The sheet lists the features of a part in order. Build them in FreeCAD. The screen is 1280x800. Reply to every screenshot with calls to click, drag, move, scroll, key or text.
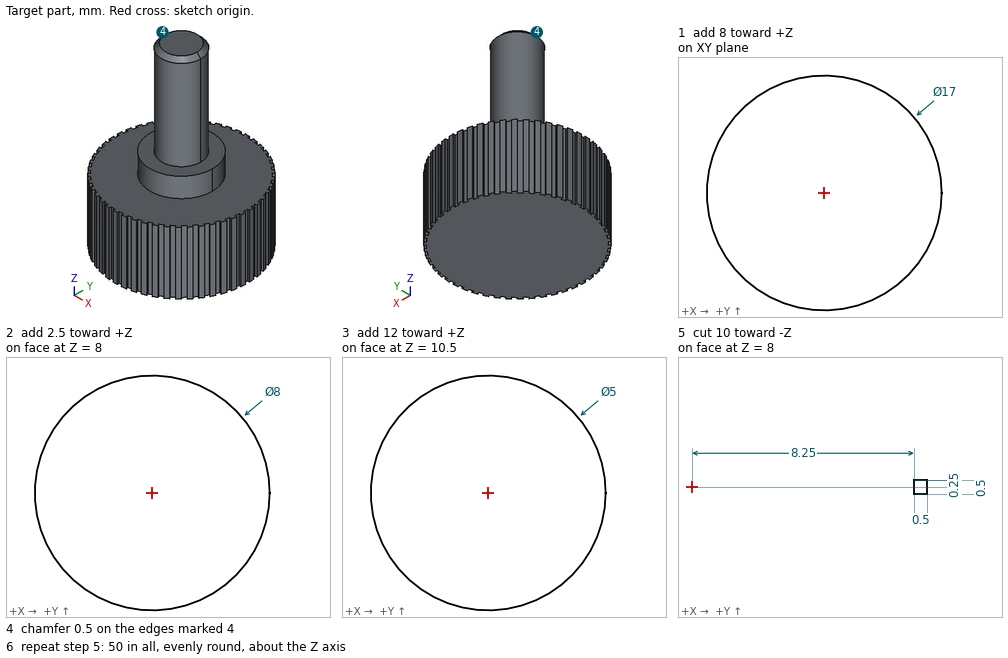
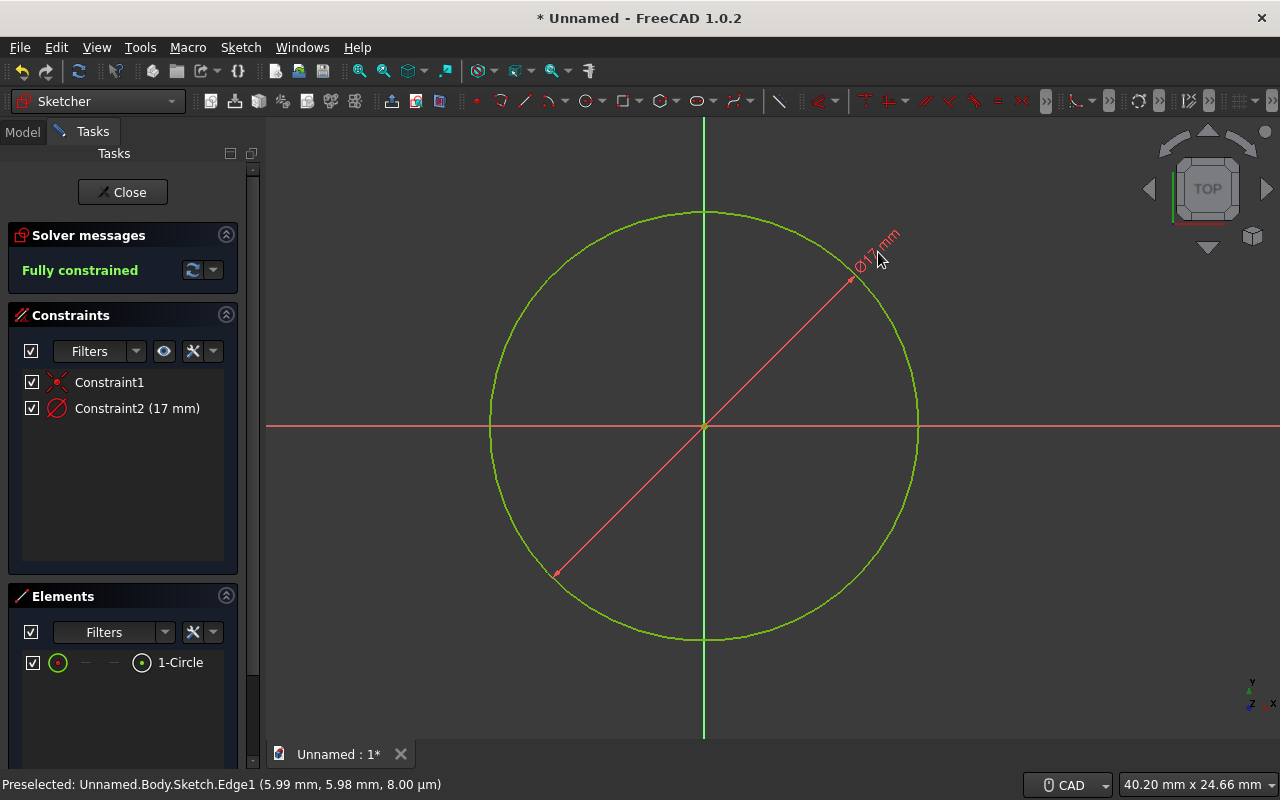
click(123, 192)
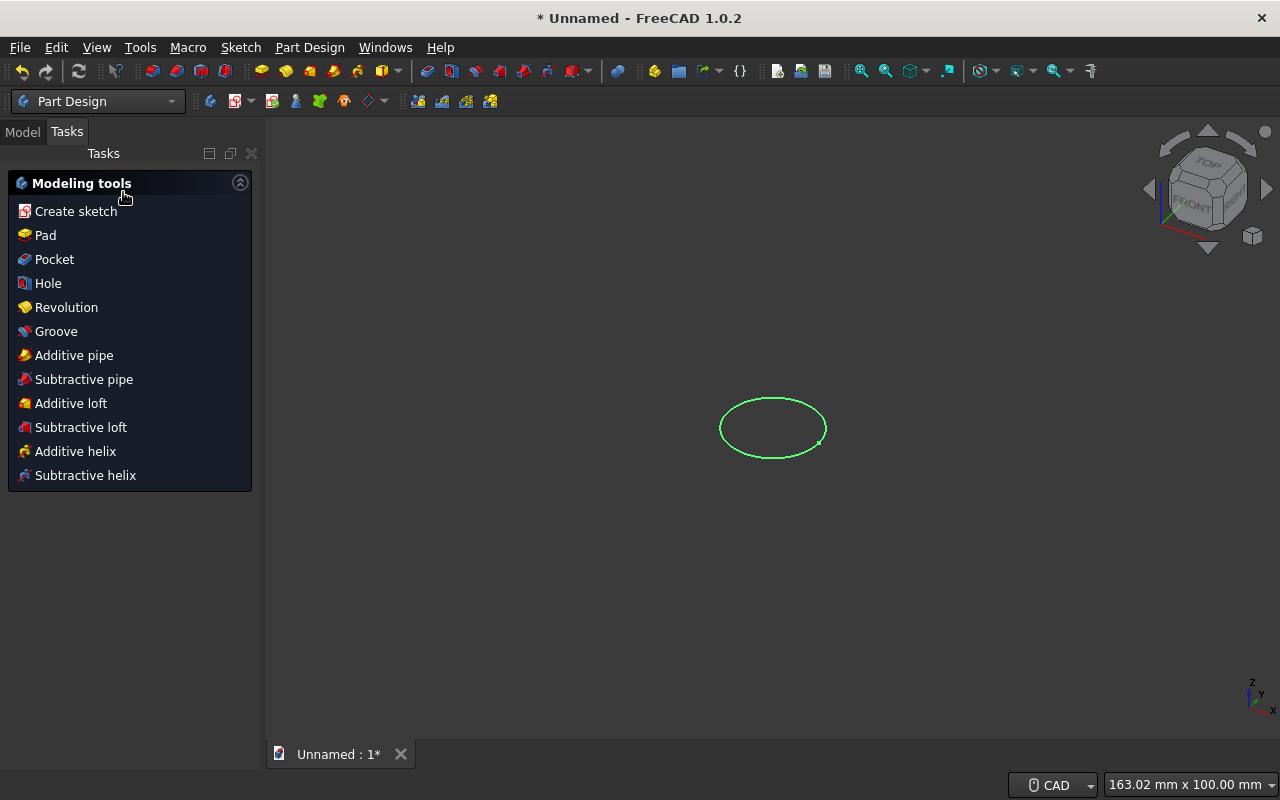
click(262, 72)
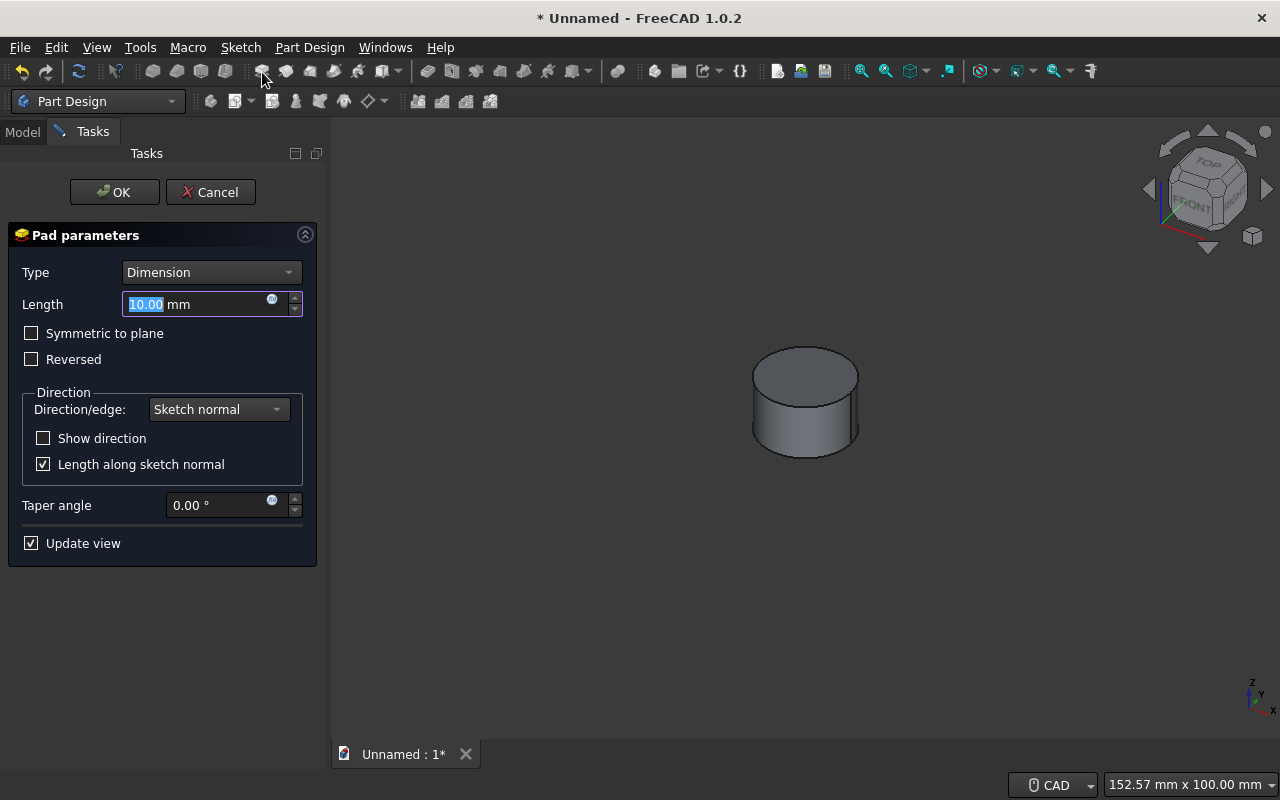
text(8)
key(Tab)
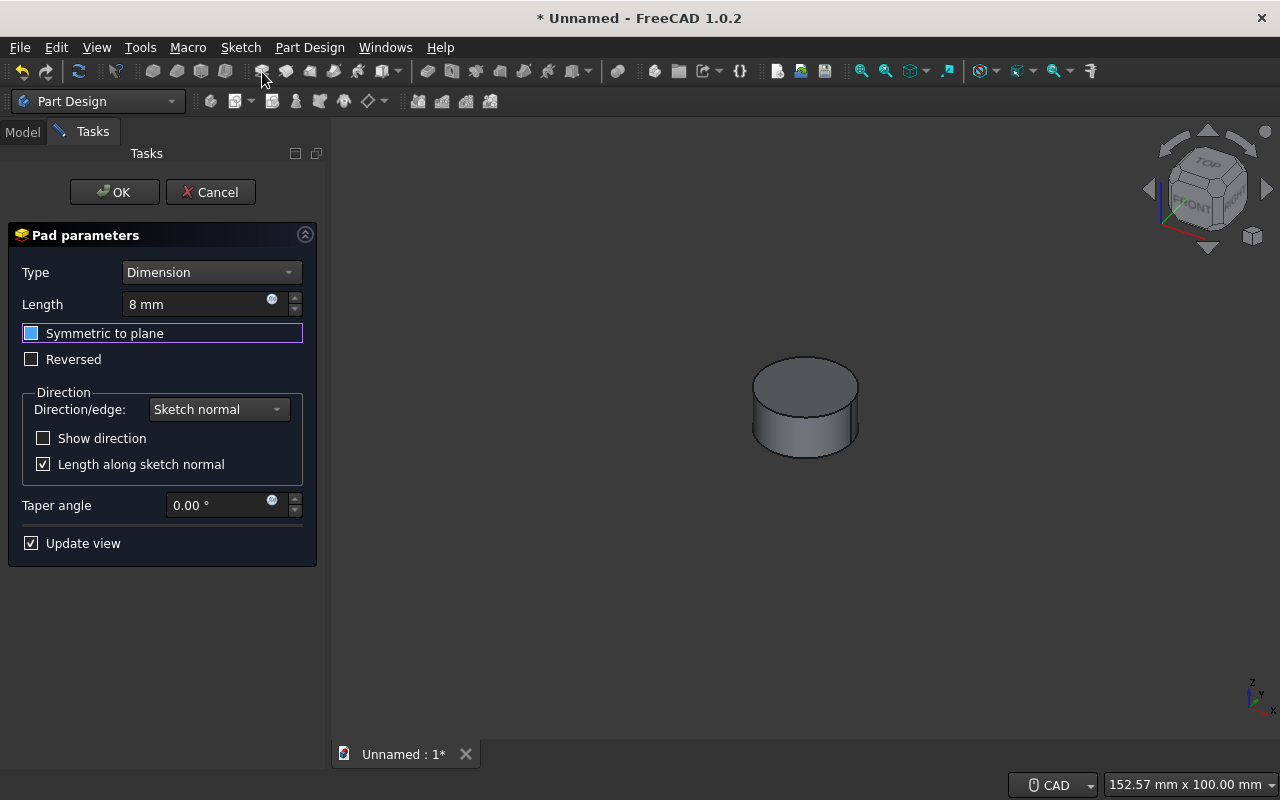
click(115, 192)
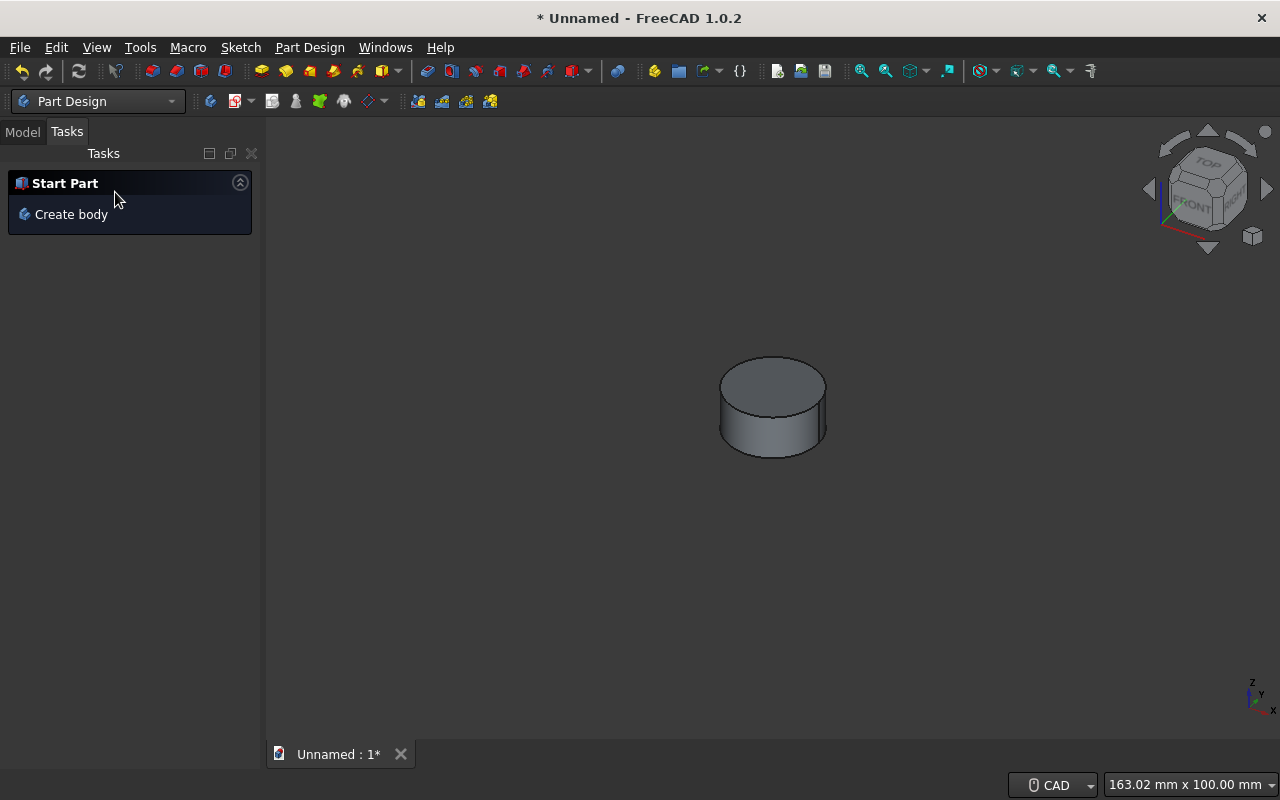
key(v)
key(f)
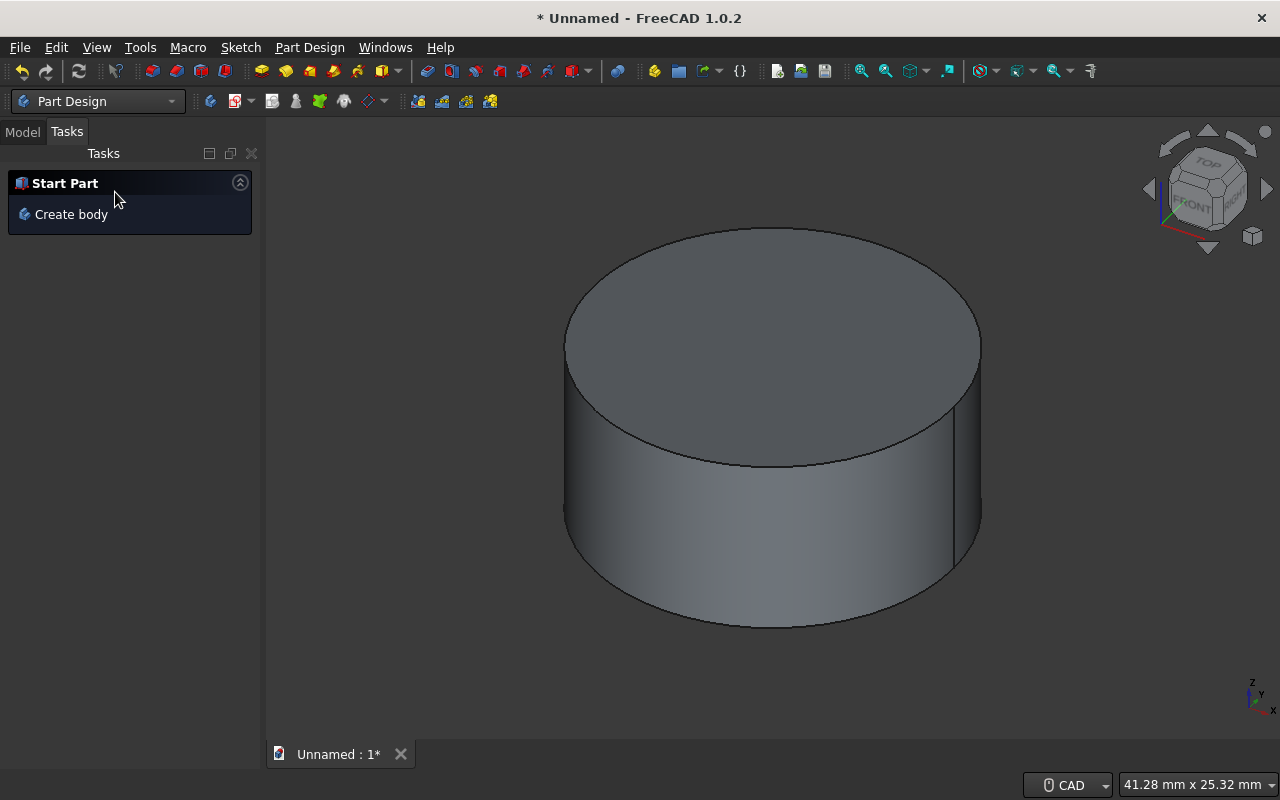
click(773, 346)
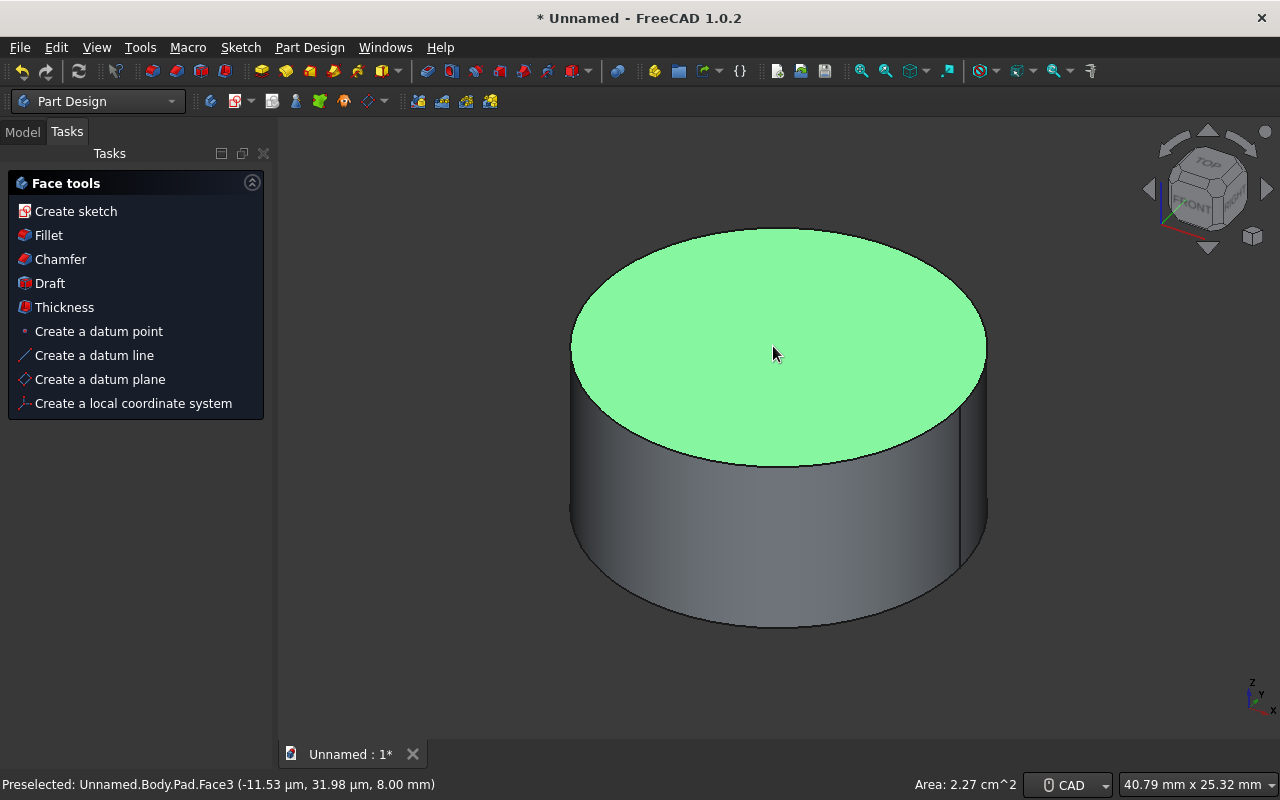
click(236, 102)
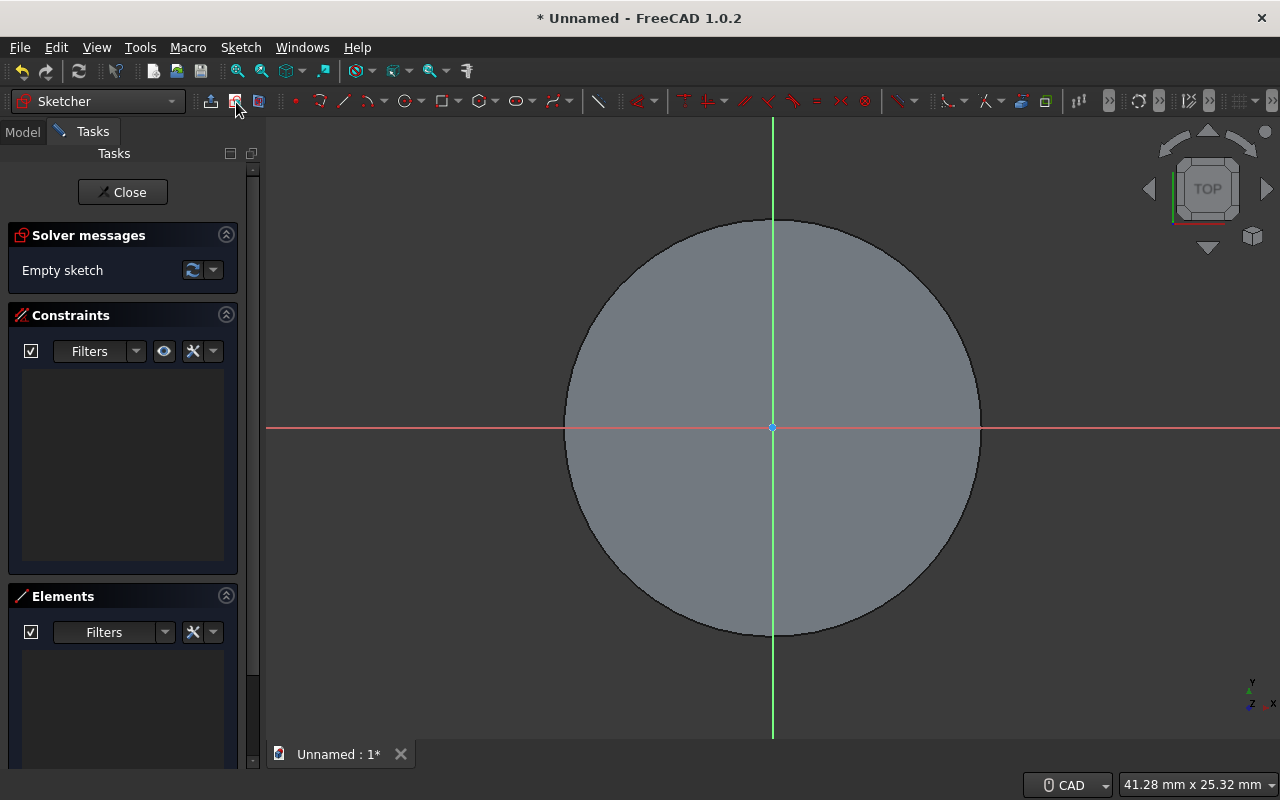
scroll(829, 428, up, 4)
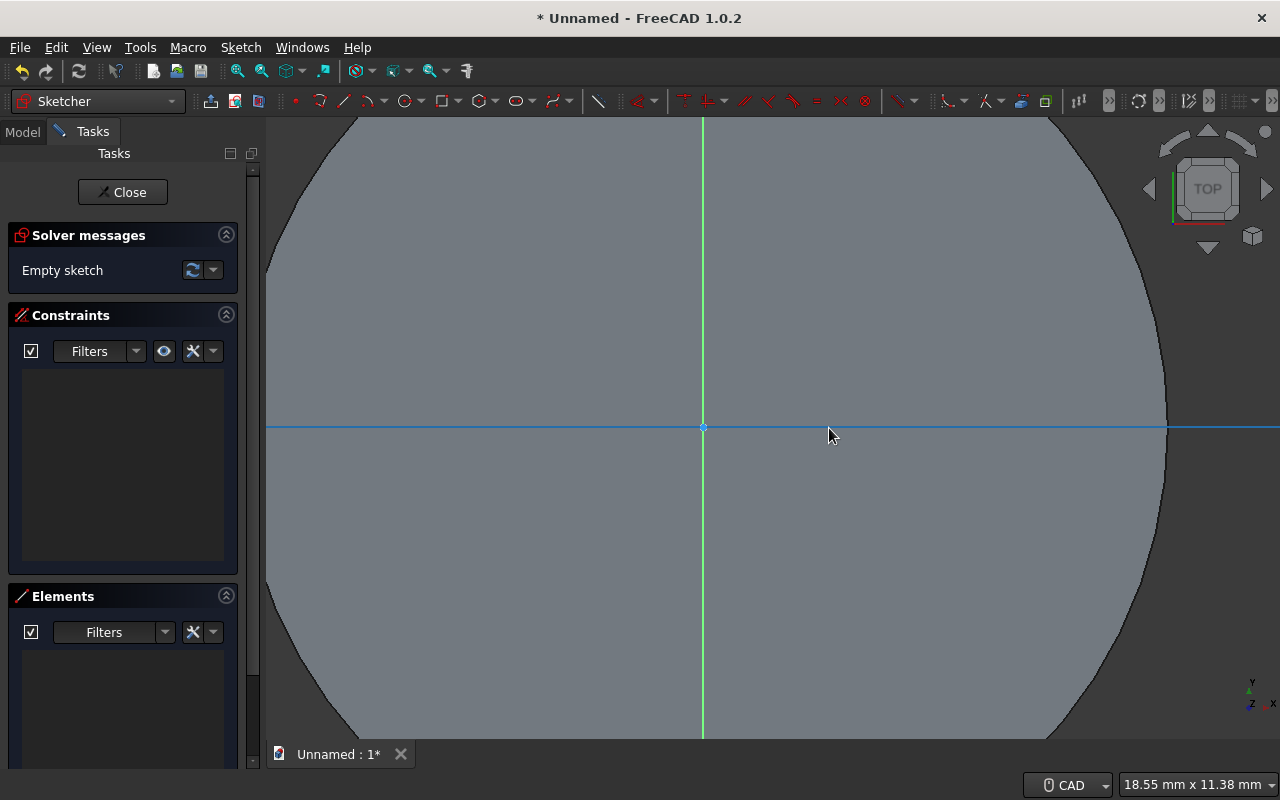
click(406, 102)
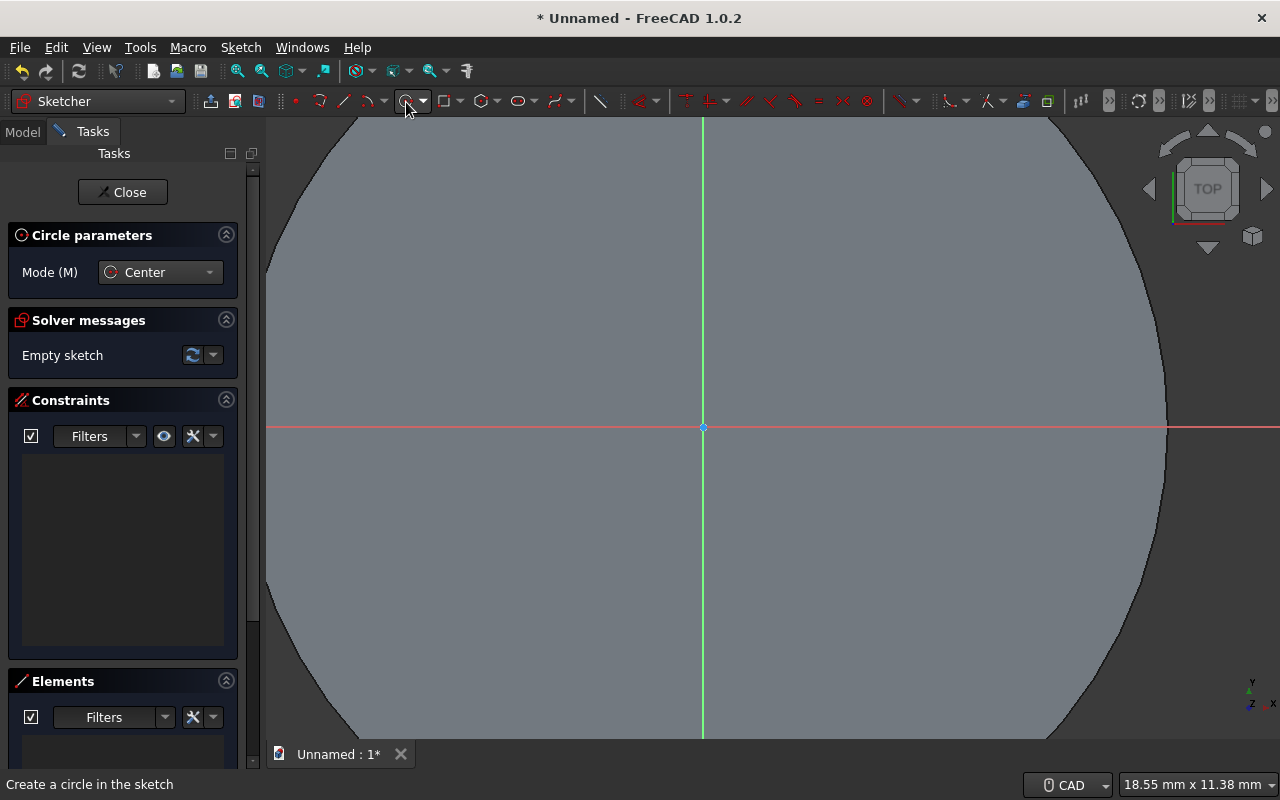
click(703, 427)
click(858, 273)
key(Escape)